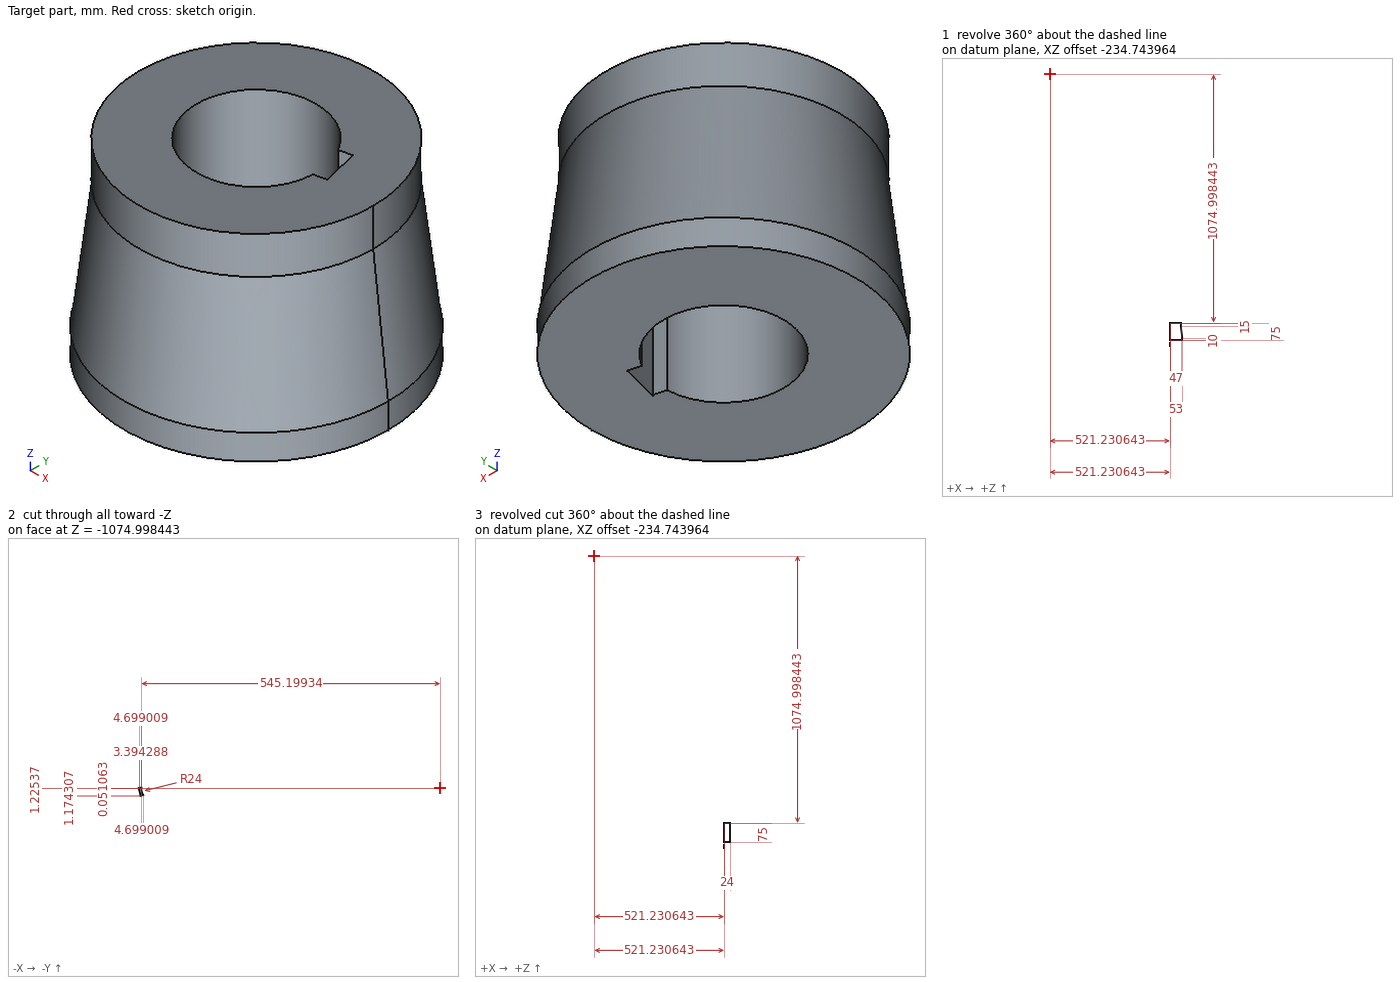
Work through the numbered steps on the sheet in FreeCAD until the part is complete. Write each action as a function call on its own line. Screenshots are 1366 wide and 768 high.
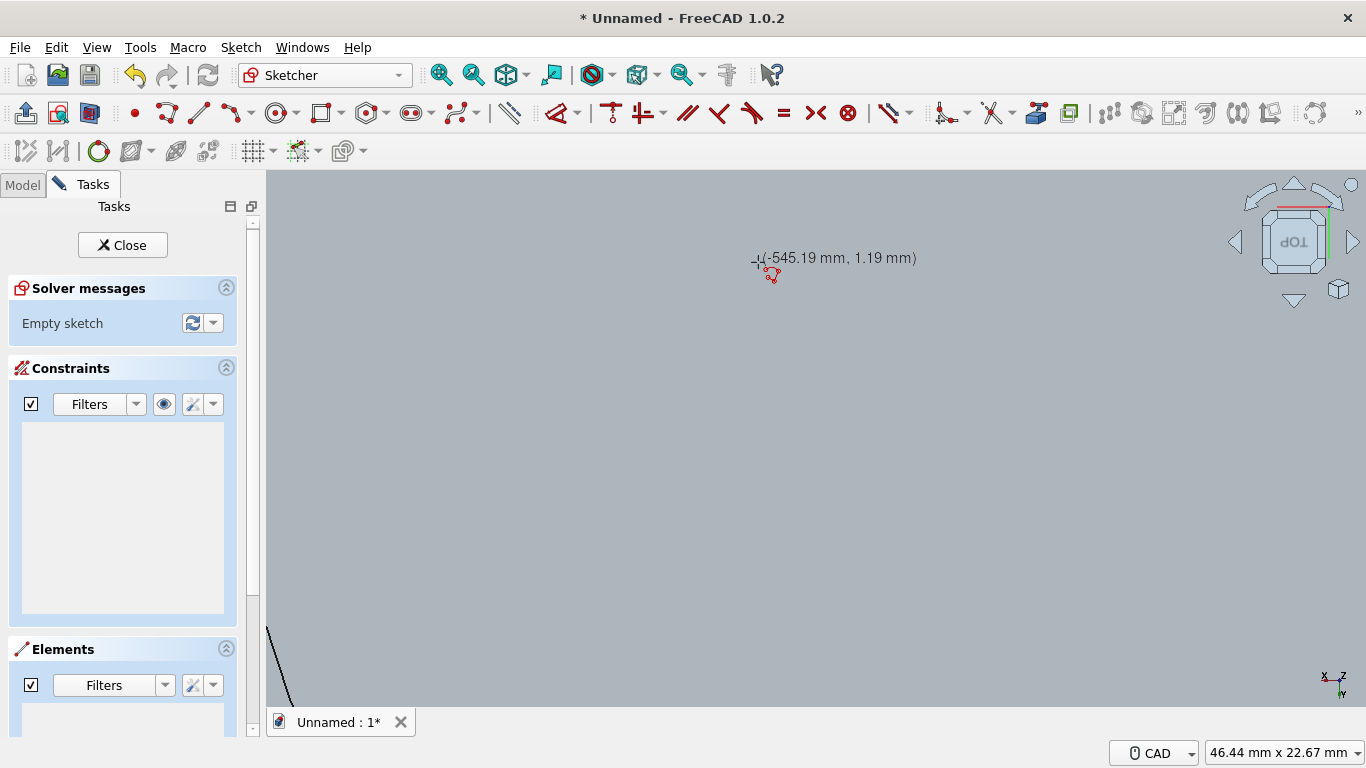
scroll(647, 290, up, 13)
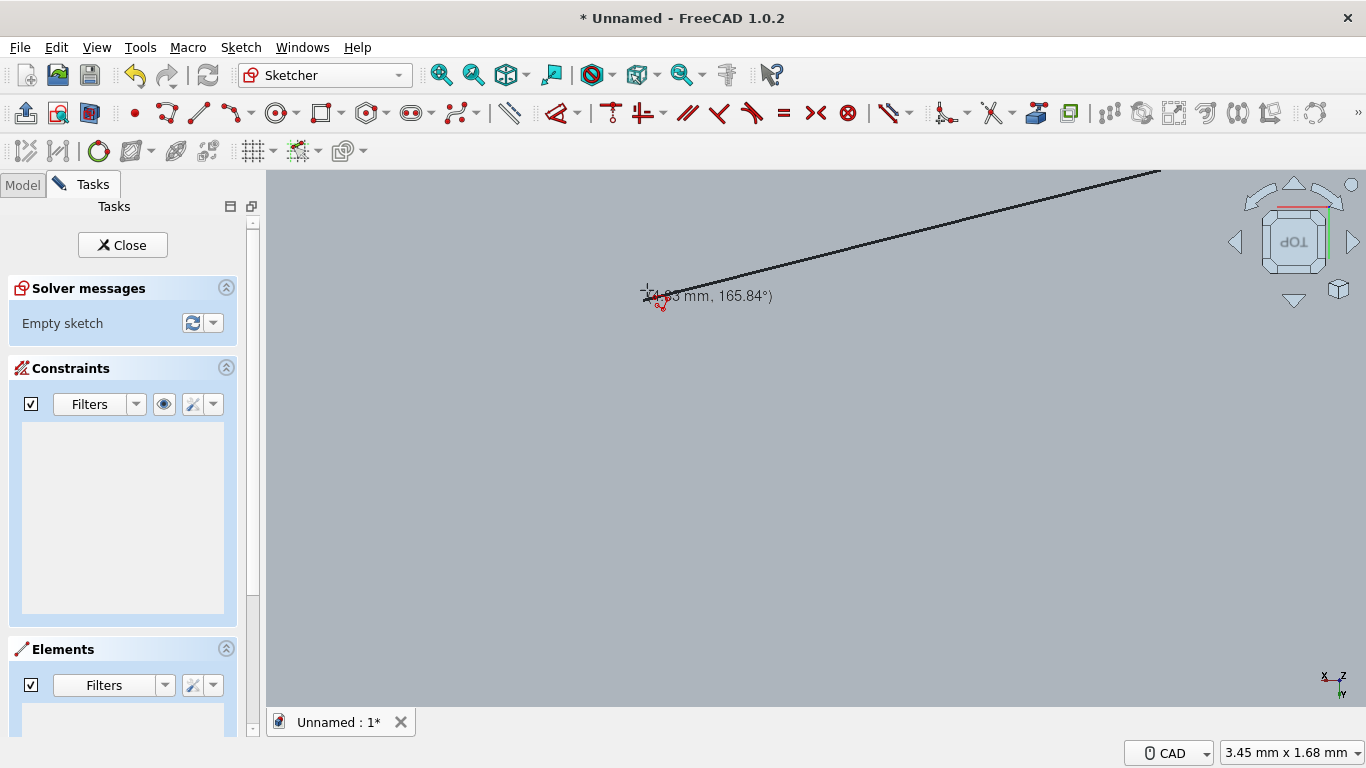
click(636, 288)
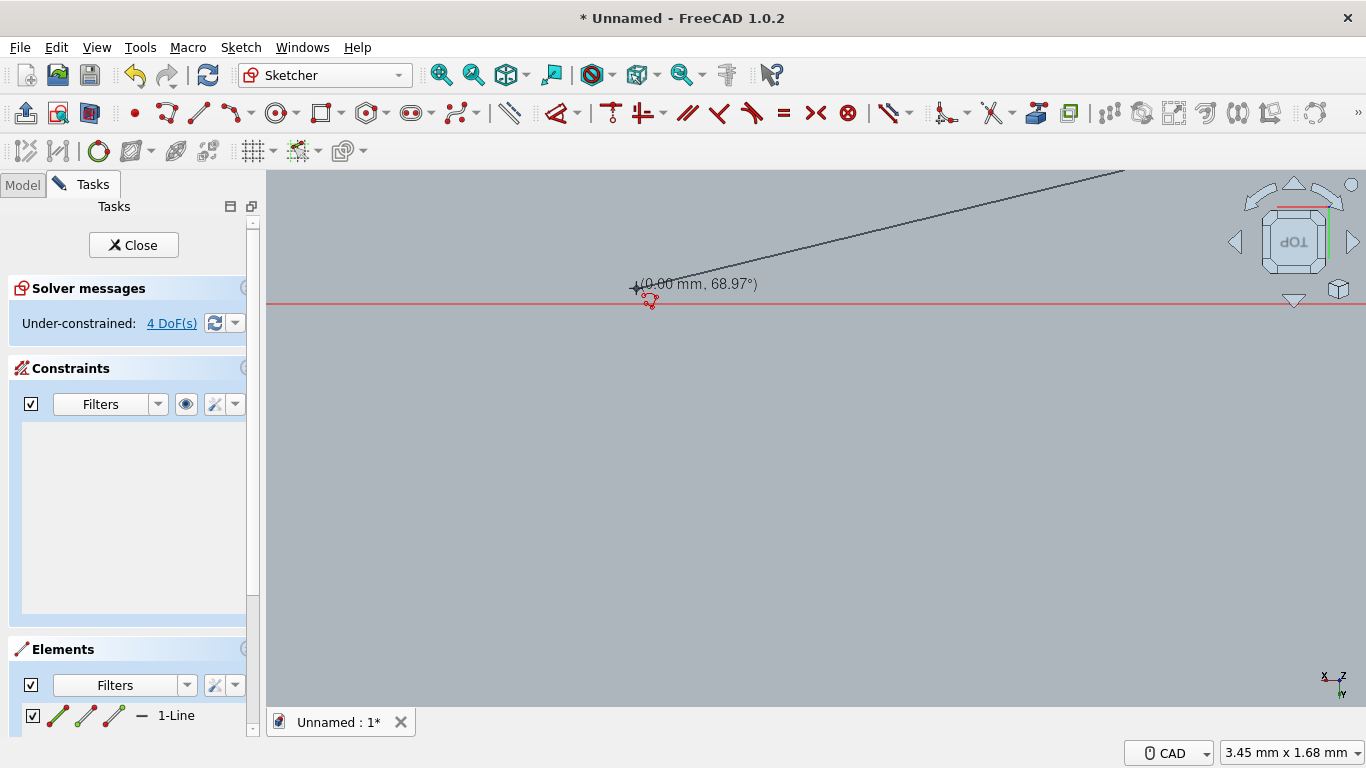
scroll(653, 292, down, 13)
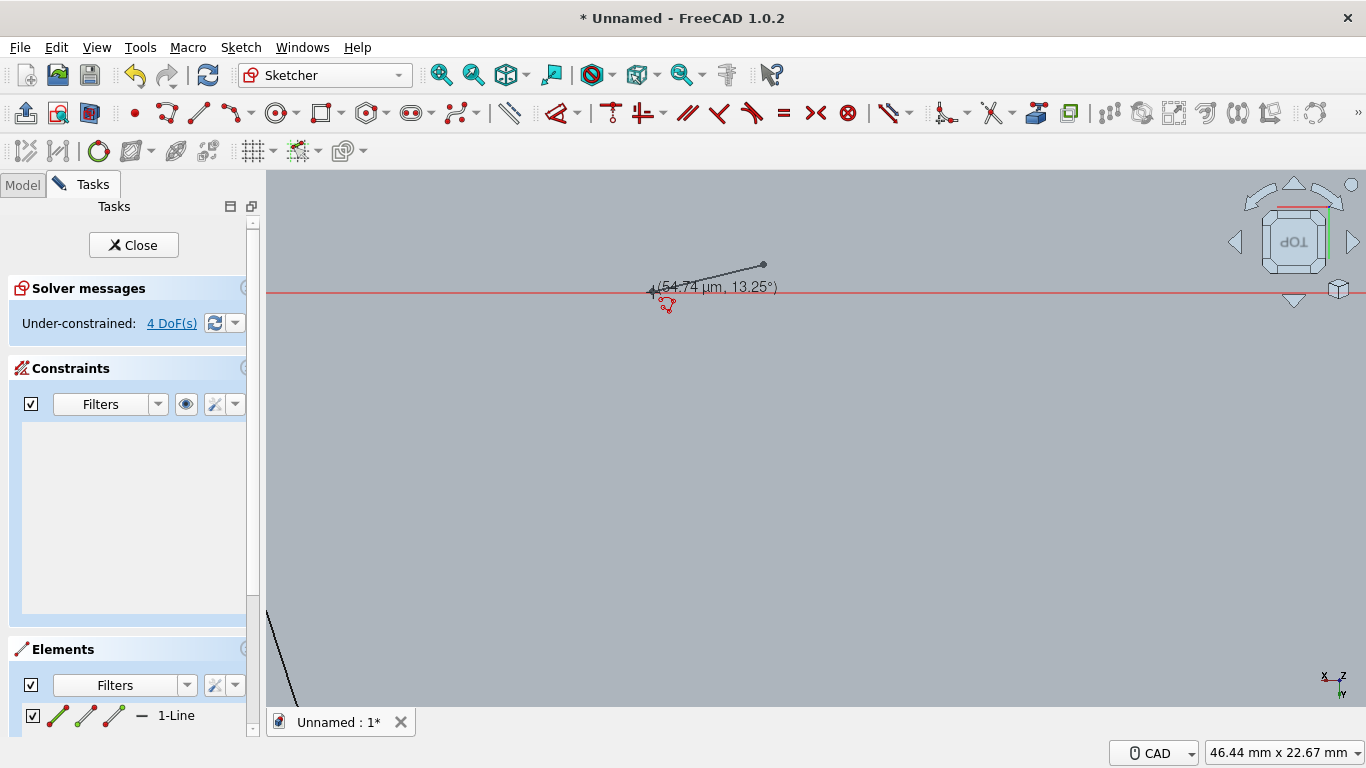
click(732, 614)
click(844, 586)
right_click(844, 586)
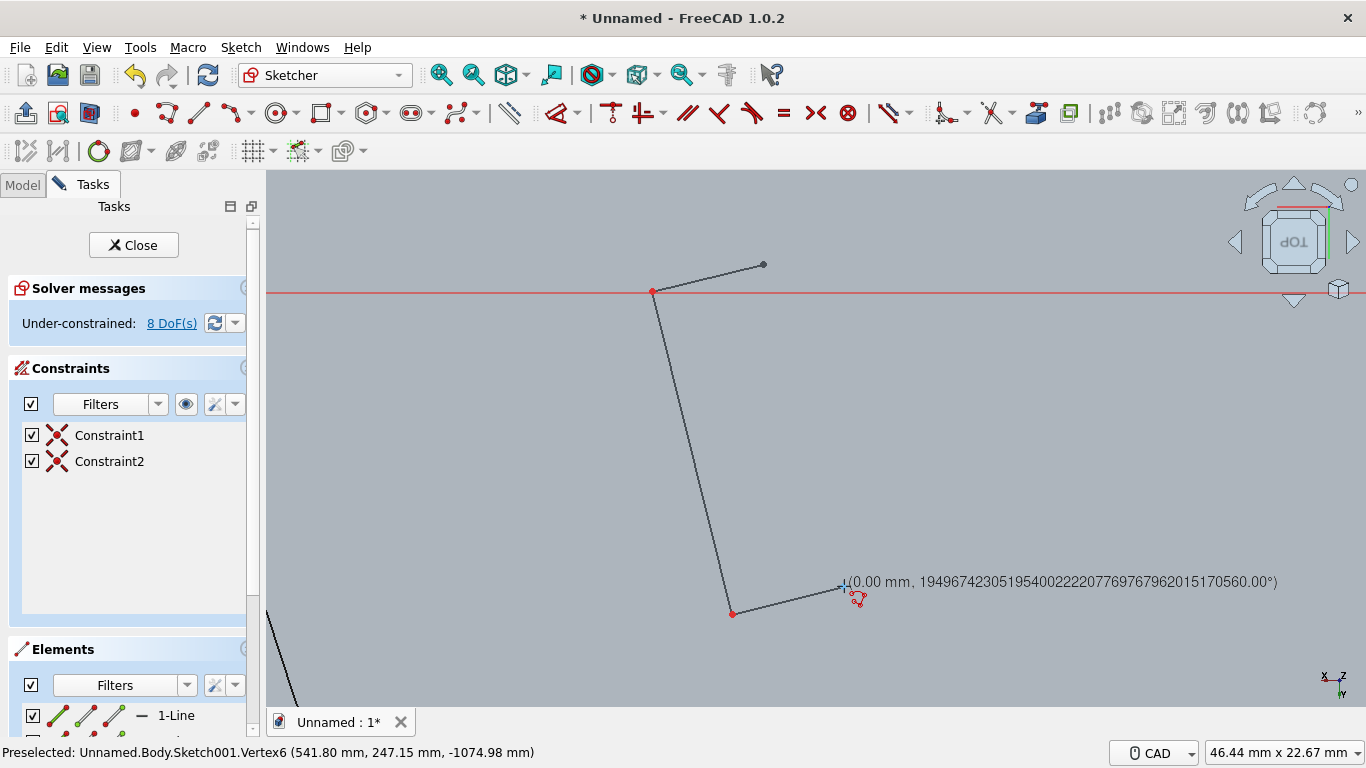
click(232, 114)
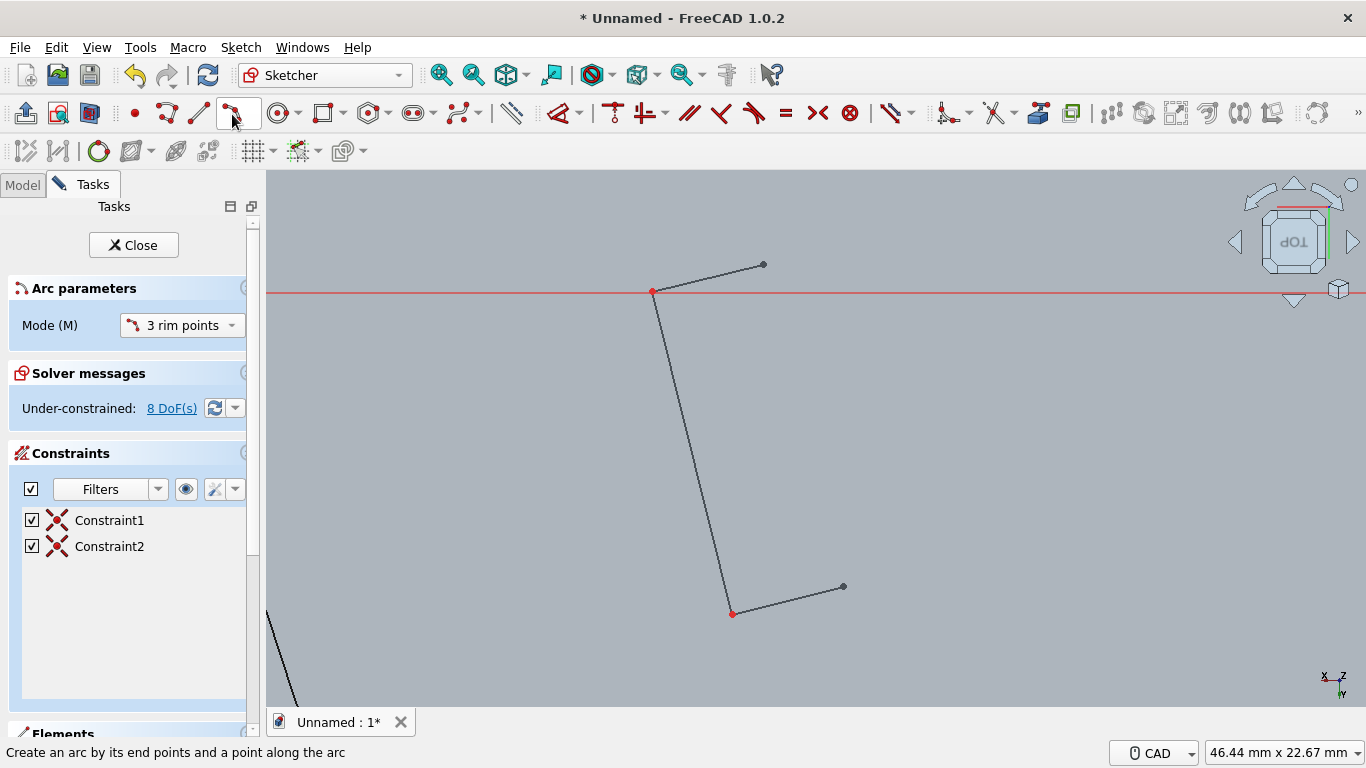
click(844, 587)
click(764, 265)
click(780, 431)
key(Escape)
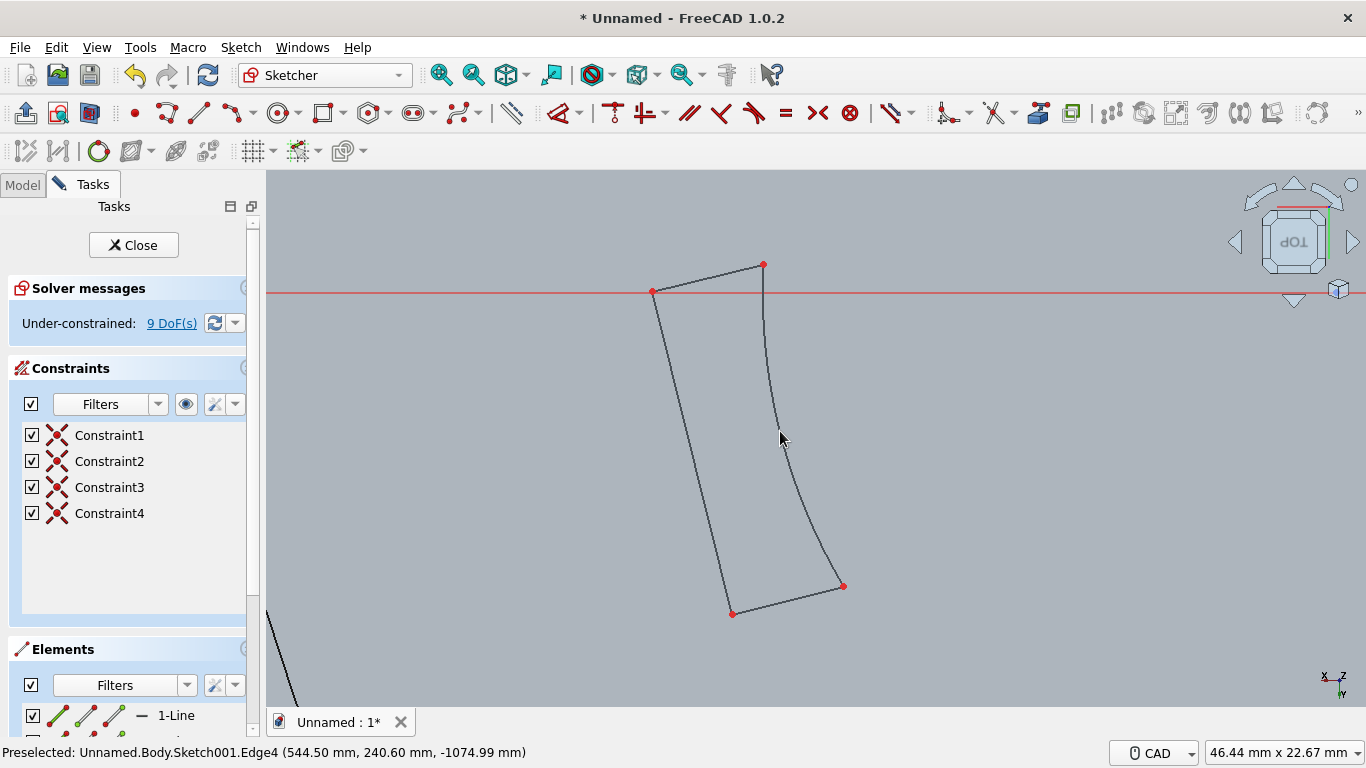
scroll(294, 437, down, 1)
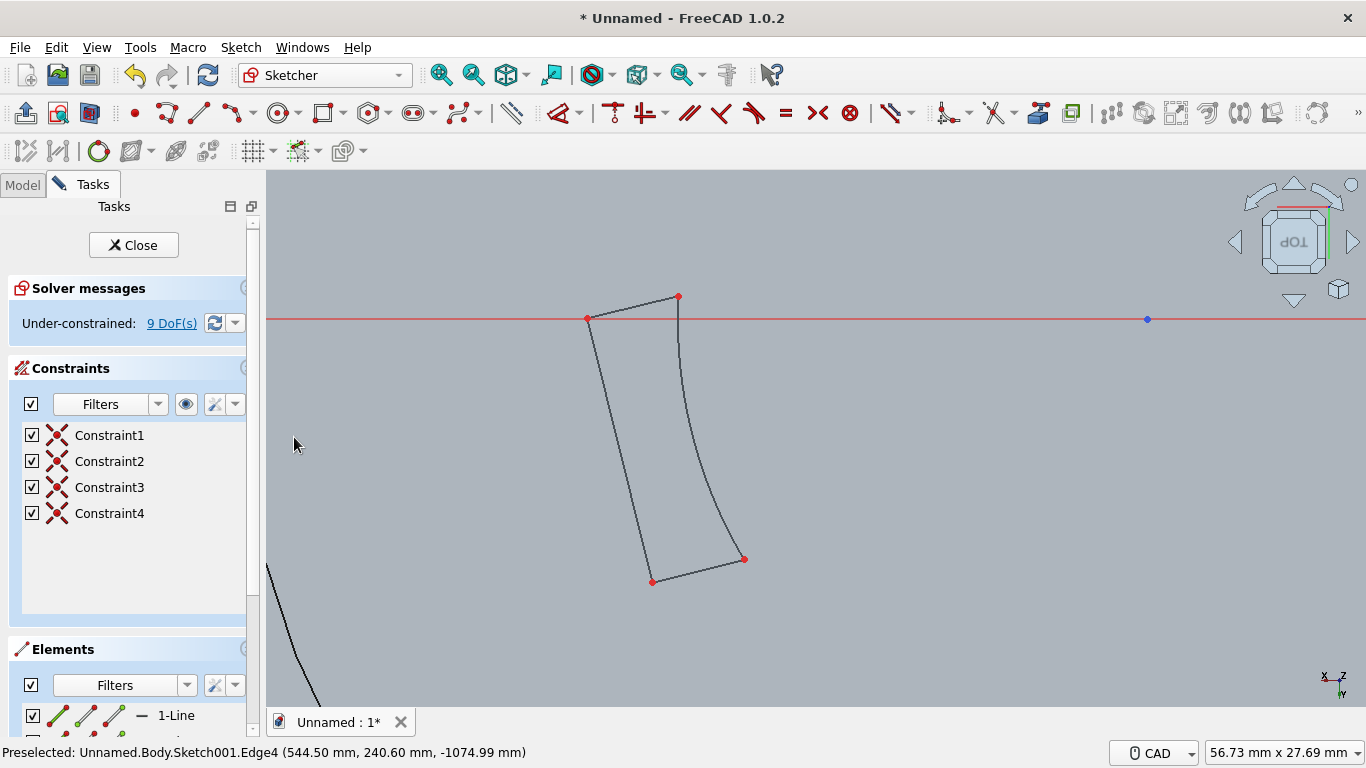
click(1148, 319)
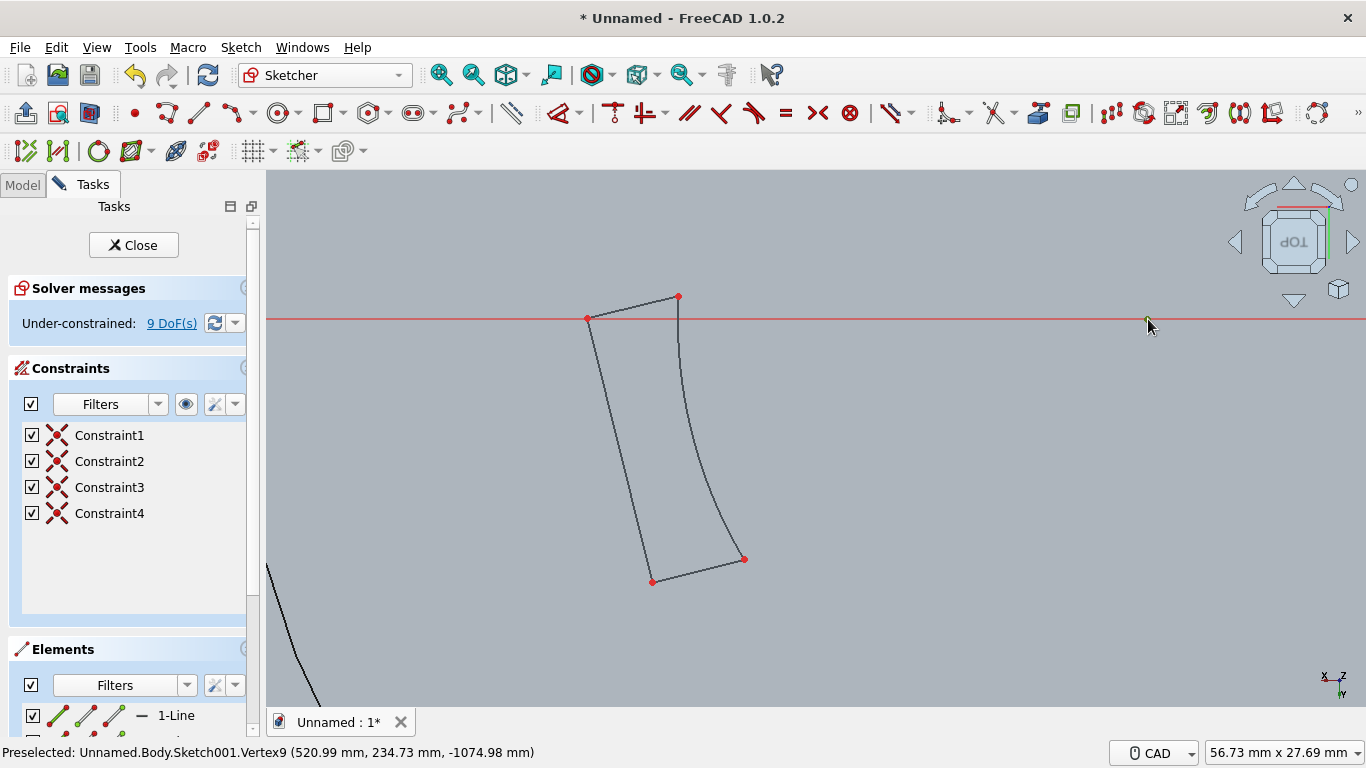
click(359, 319)